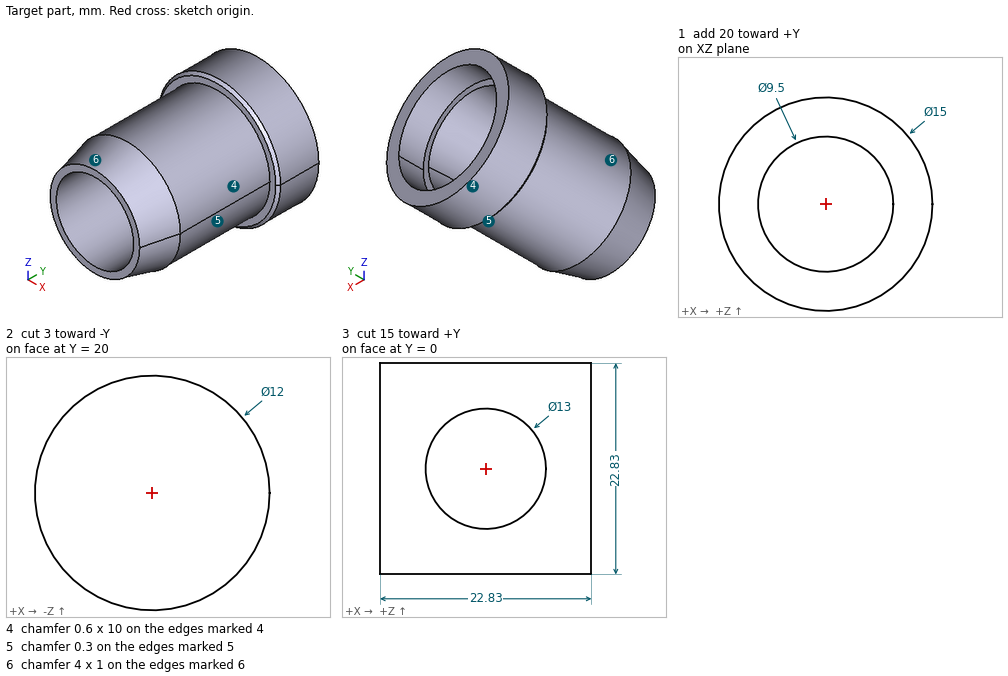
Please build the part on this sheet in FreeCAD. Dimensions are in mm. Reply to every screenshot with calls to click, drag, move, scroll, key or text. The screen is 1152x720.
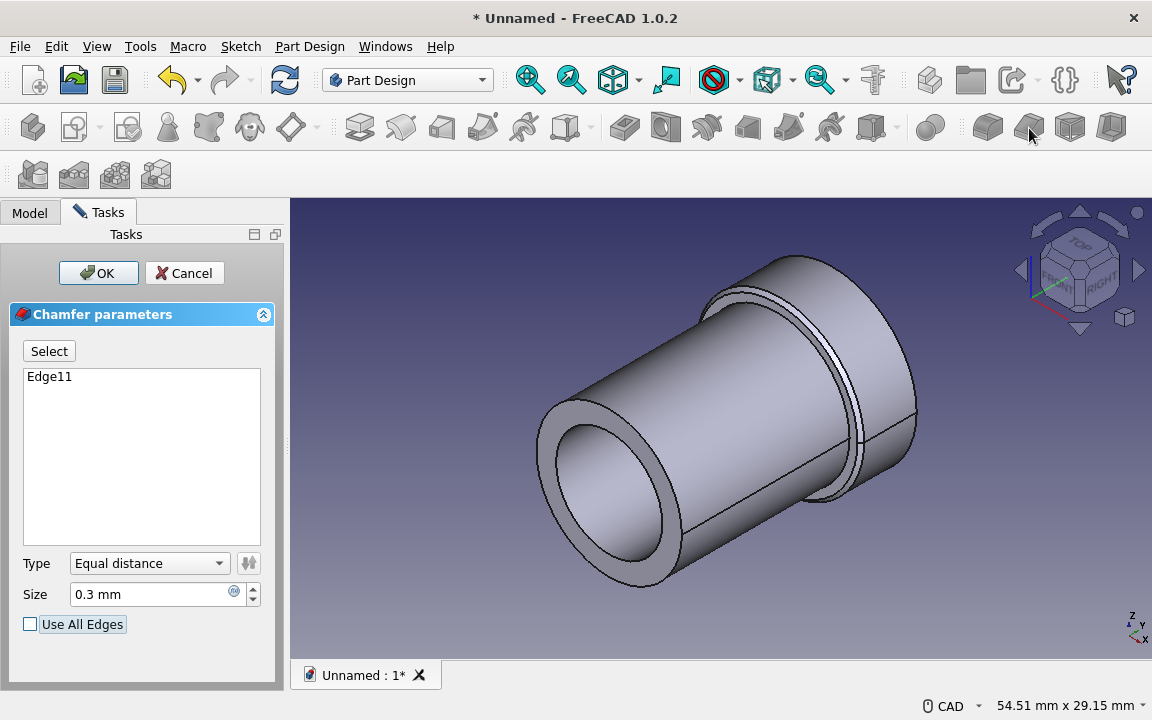
click(99, 273)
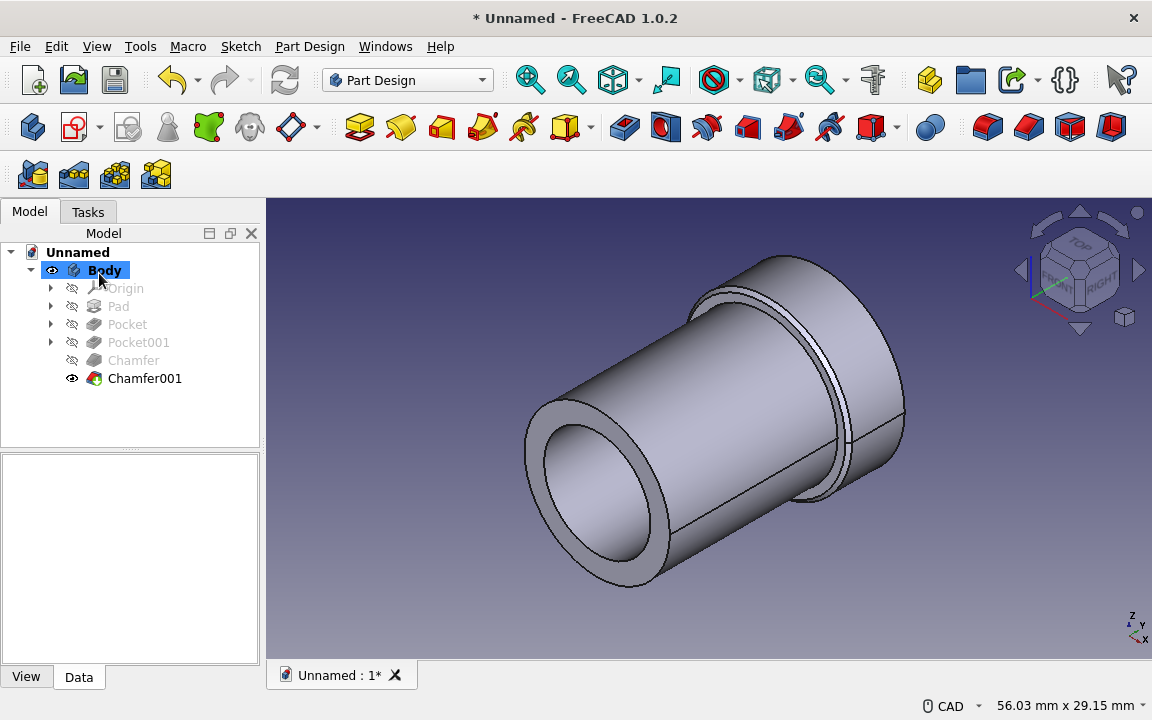
click(575, 399)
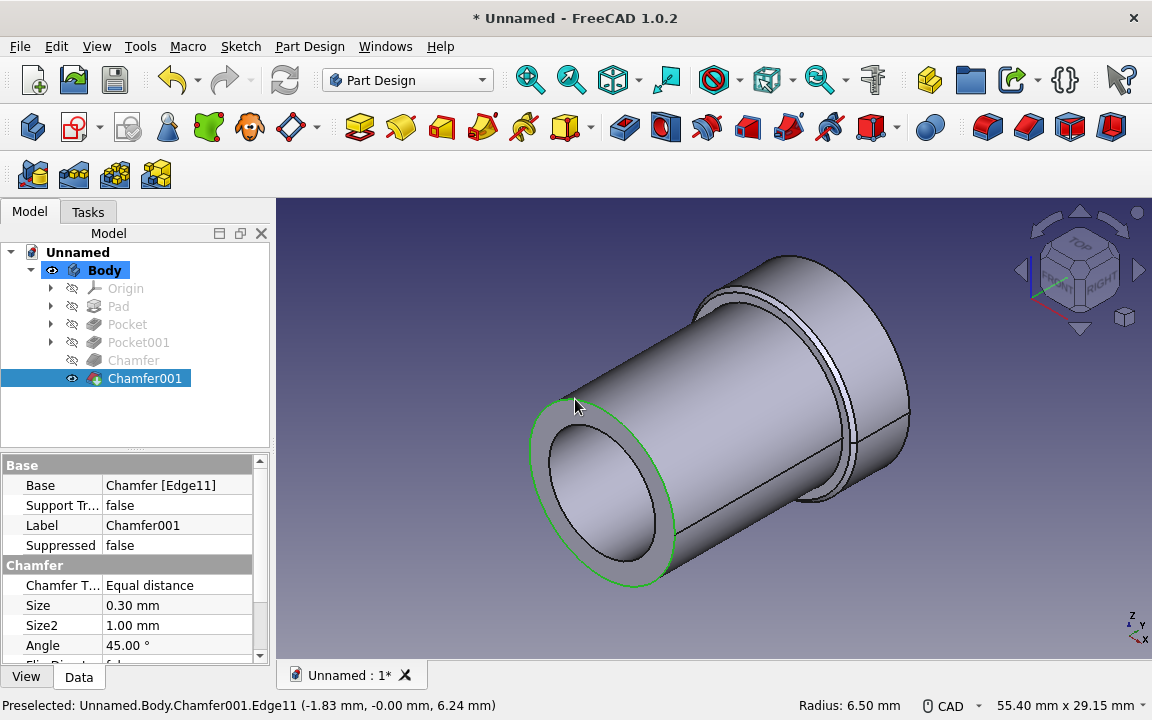
click(1029, 128)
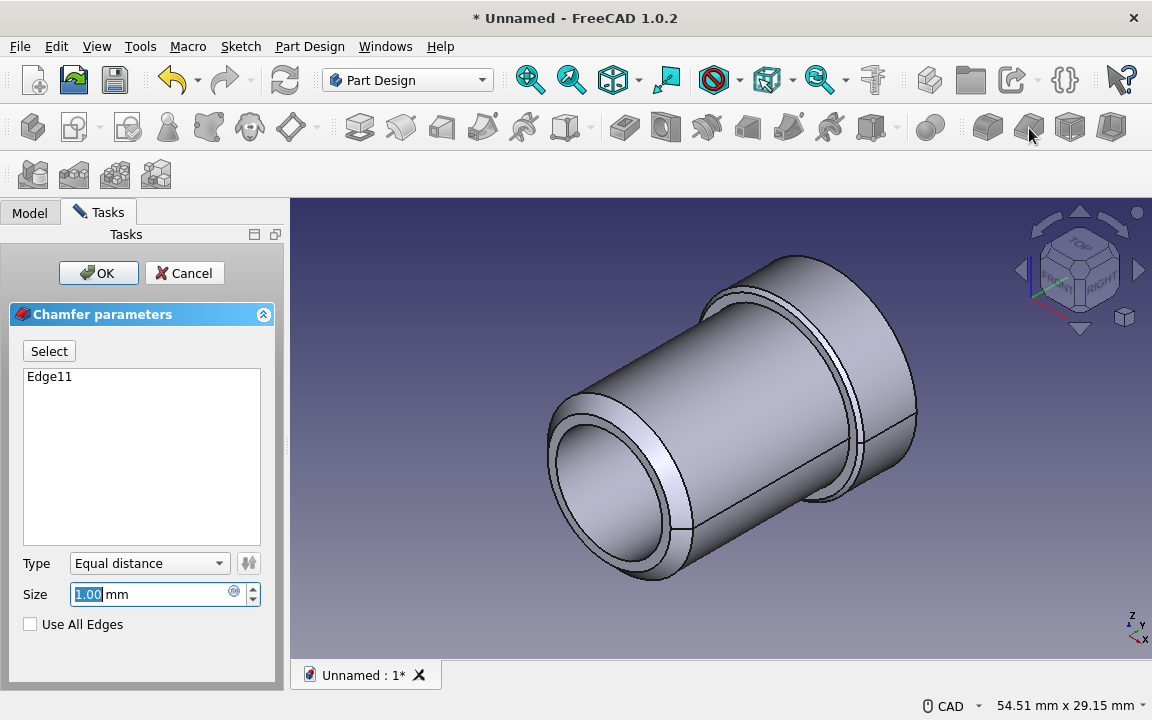
text(4)
key(Tab)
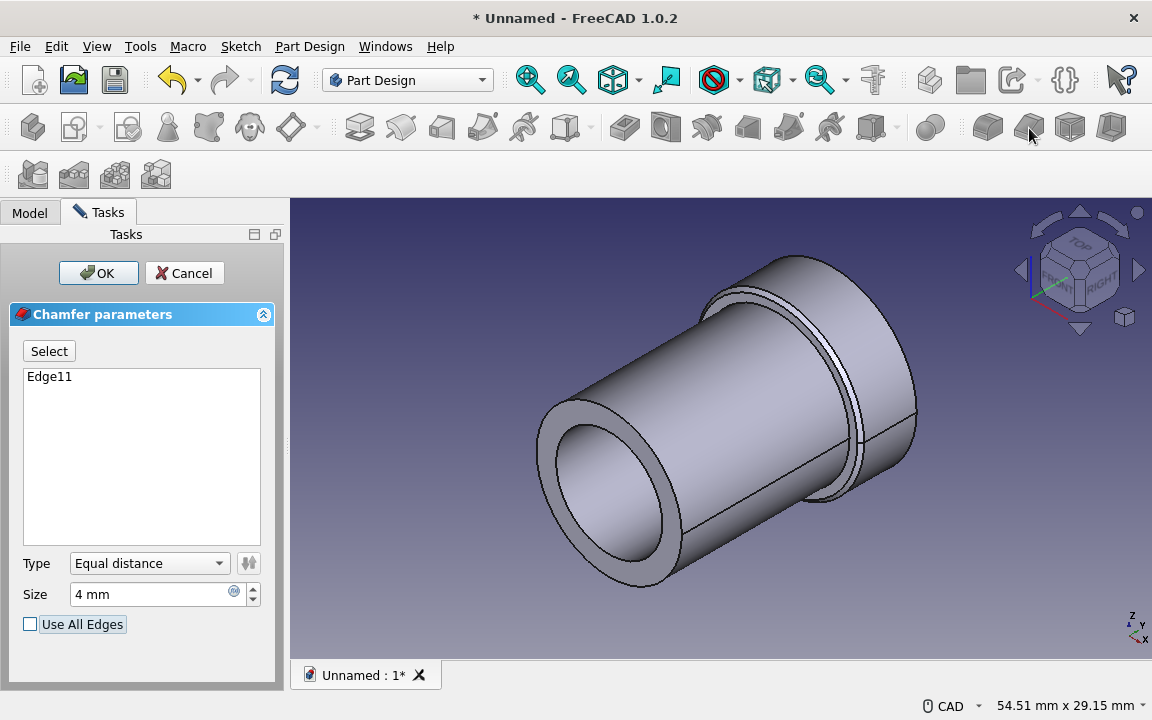
click(150, 564)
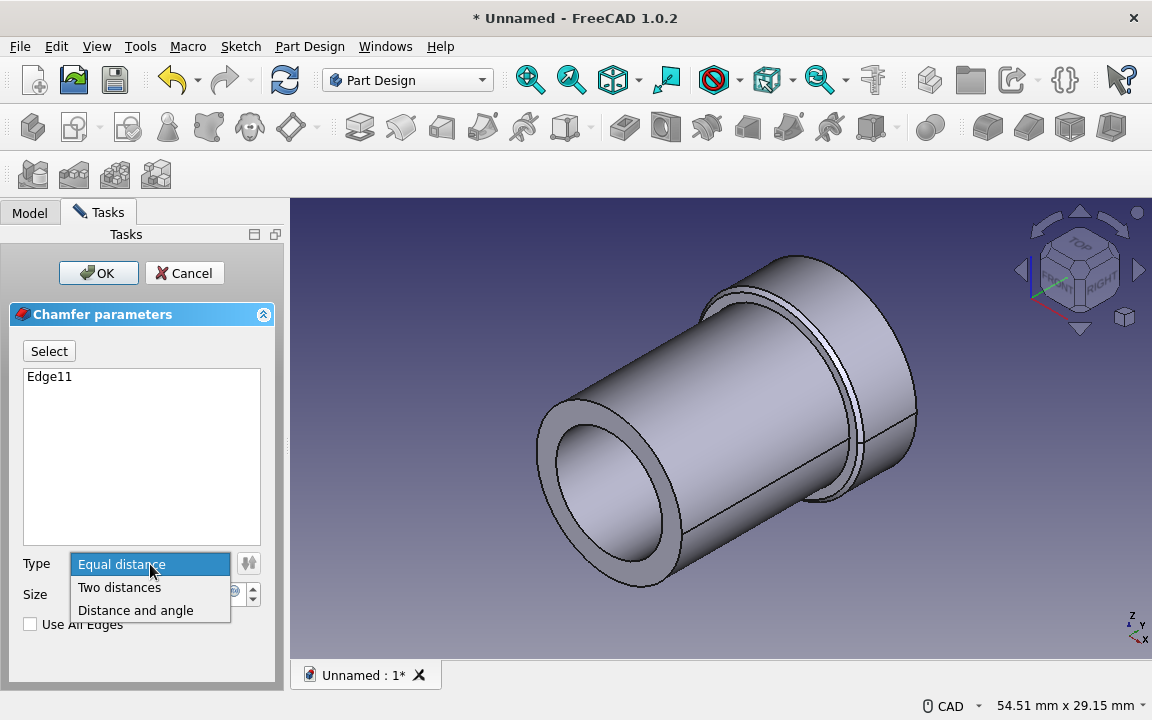
click(148, 588)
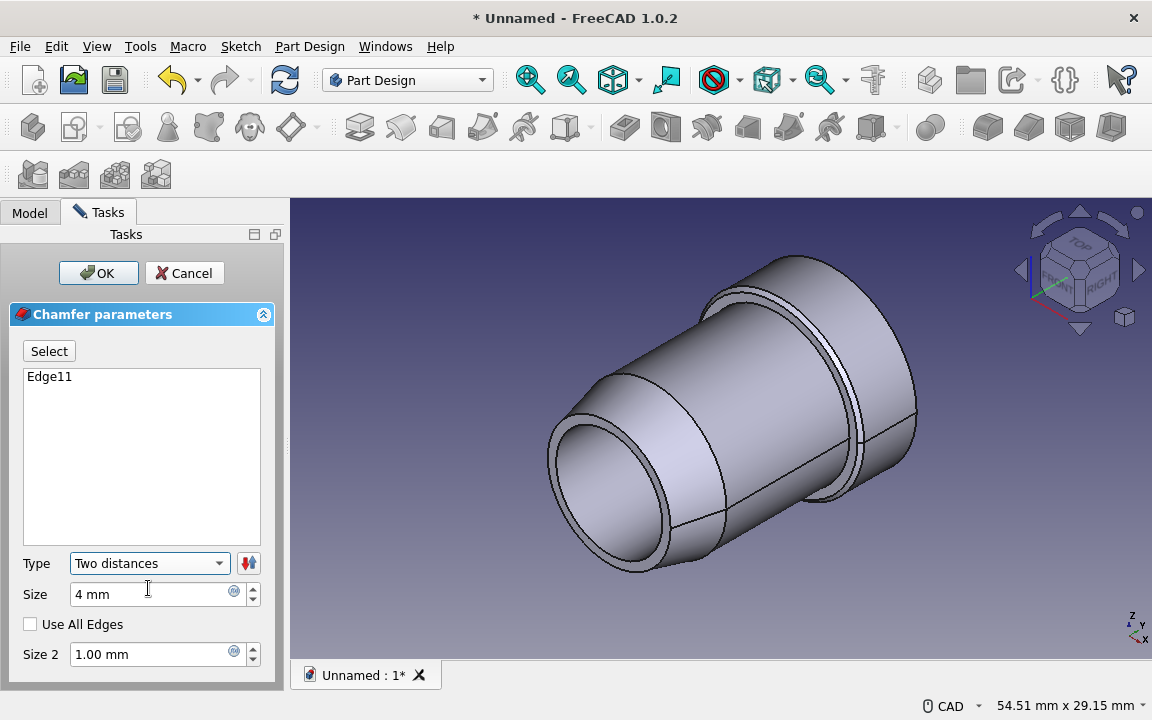
triple_click(158, 654)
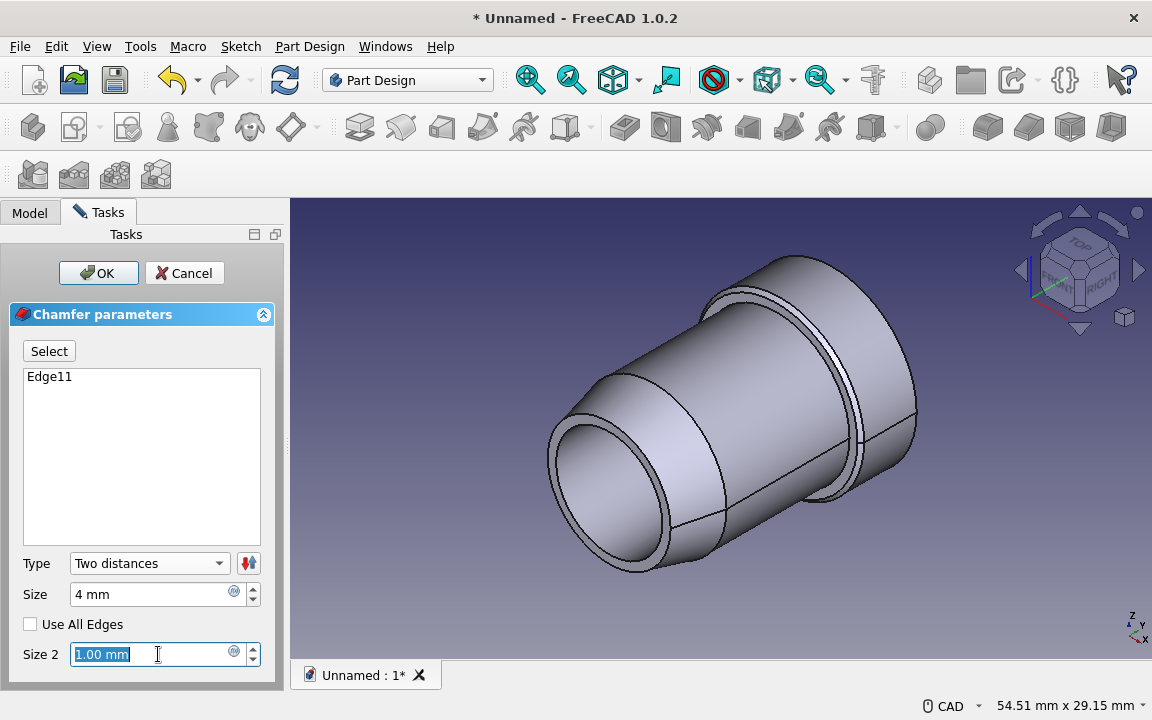
text(1)
key(Tab)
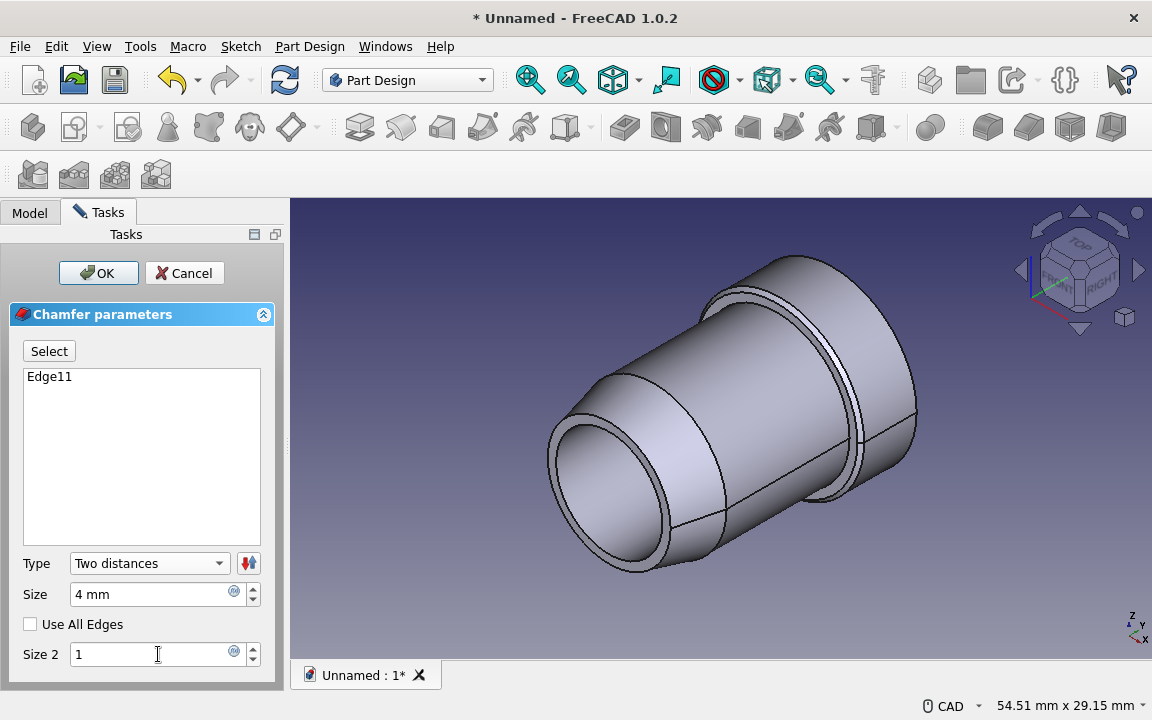
click(99, 273)